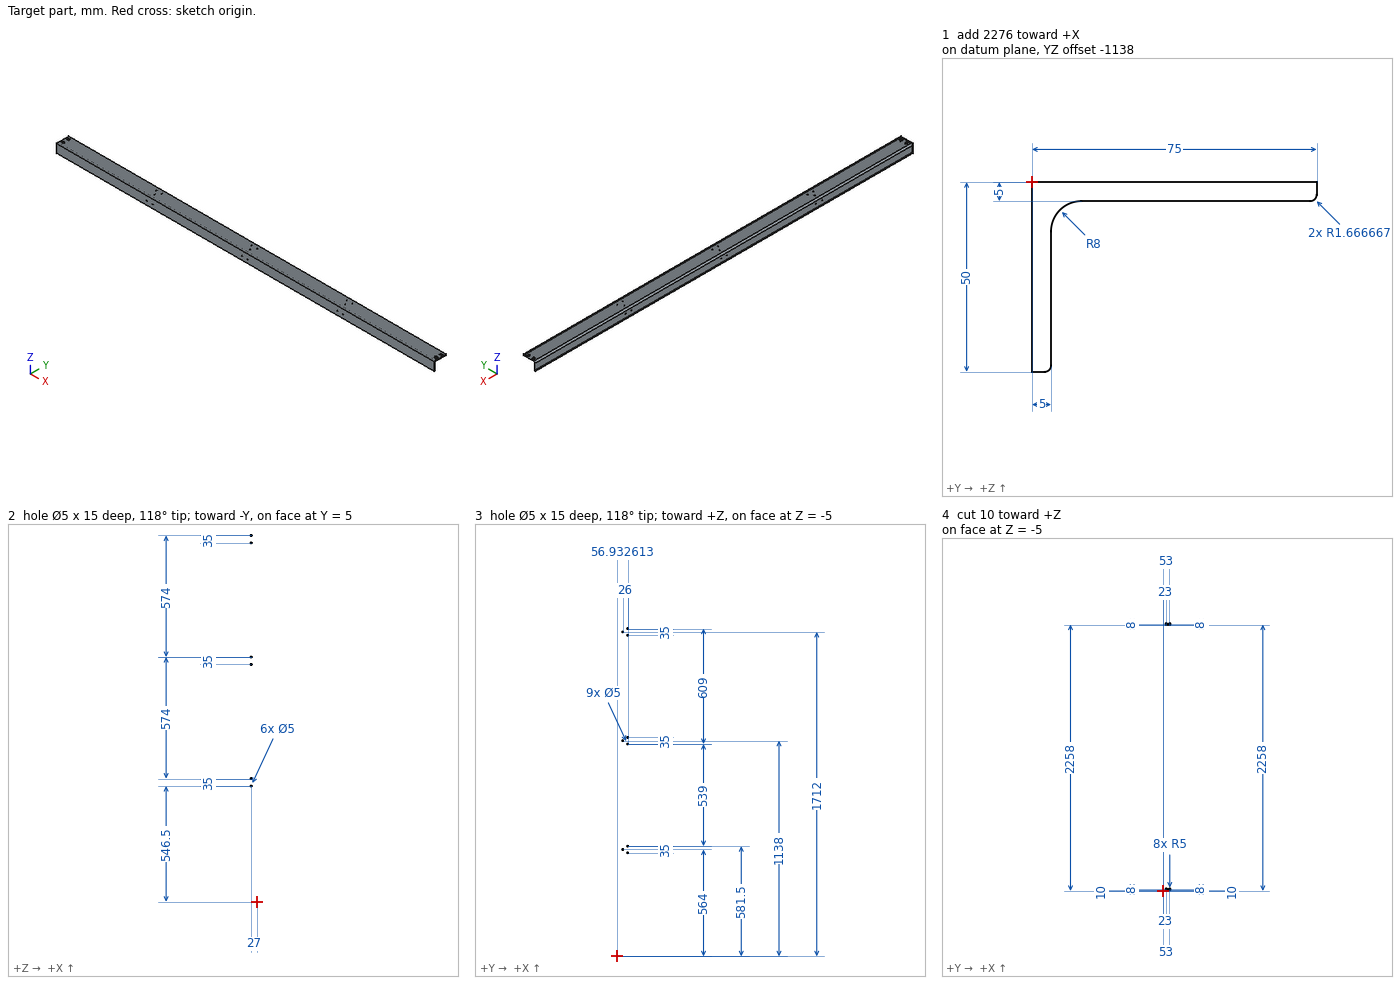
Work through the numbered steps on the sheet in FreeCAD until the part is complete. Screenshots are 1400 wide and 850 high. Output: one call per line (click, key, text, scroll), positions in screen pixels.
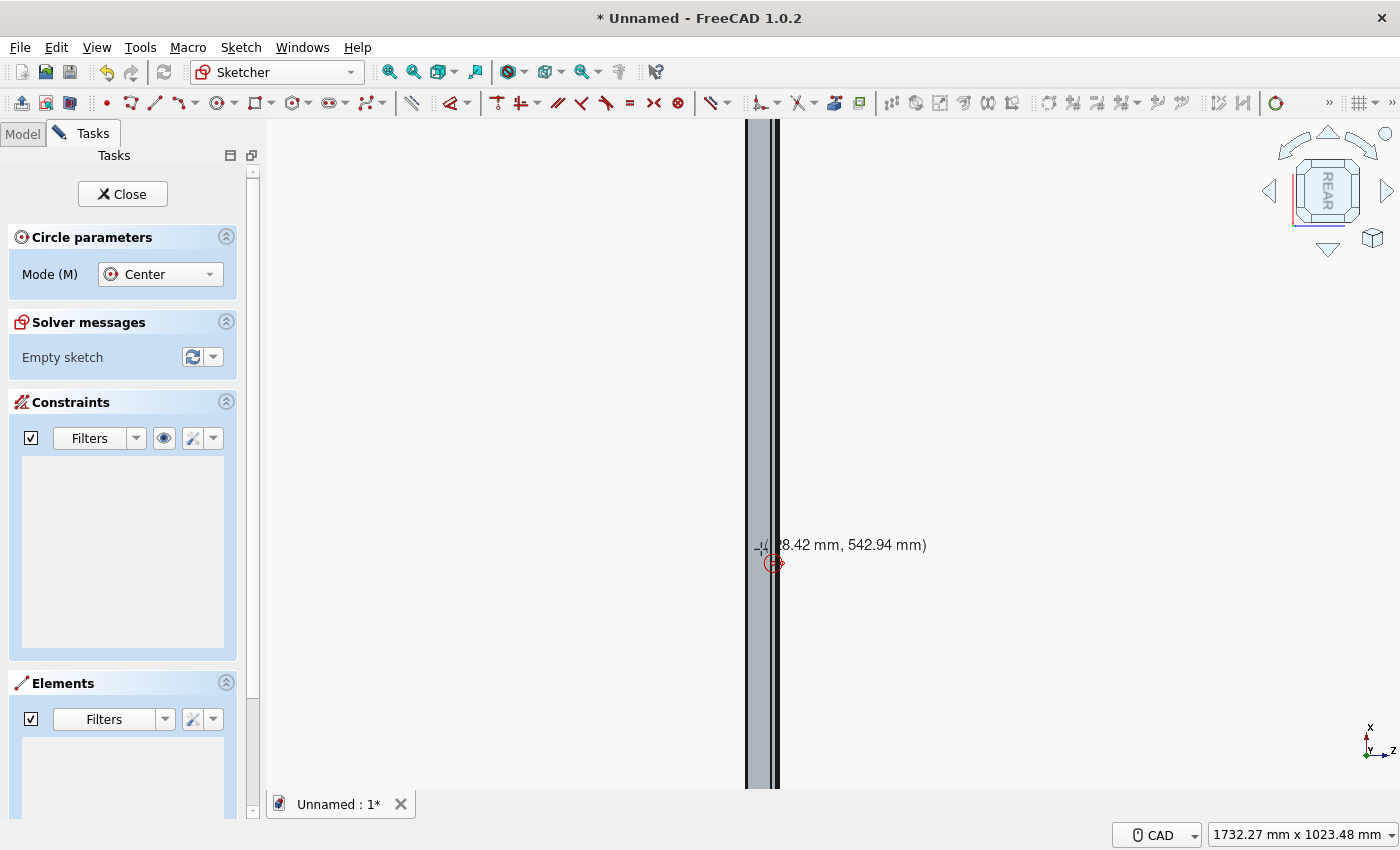
click(761, 548)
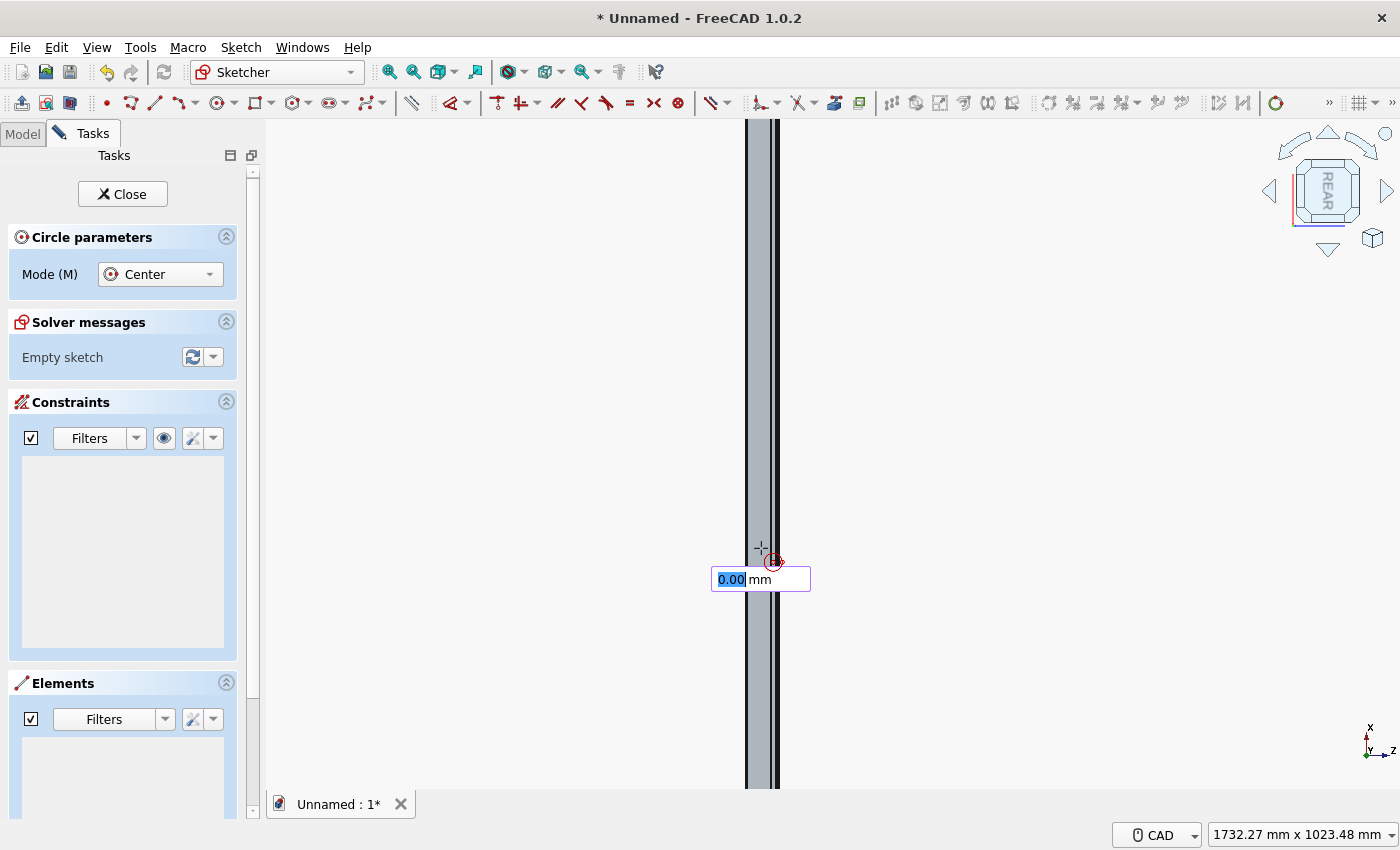
scroll(763, 547, up, 12)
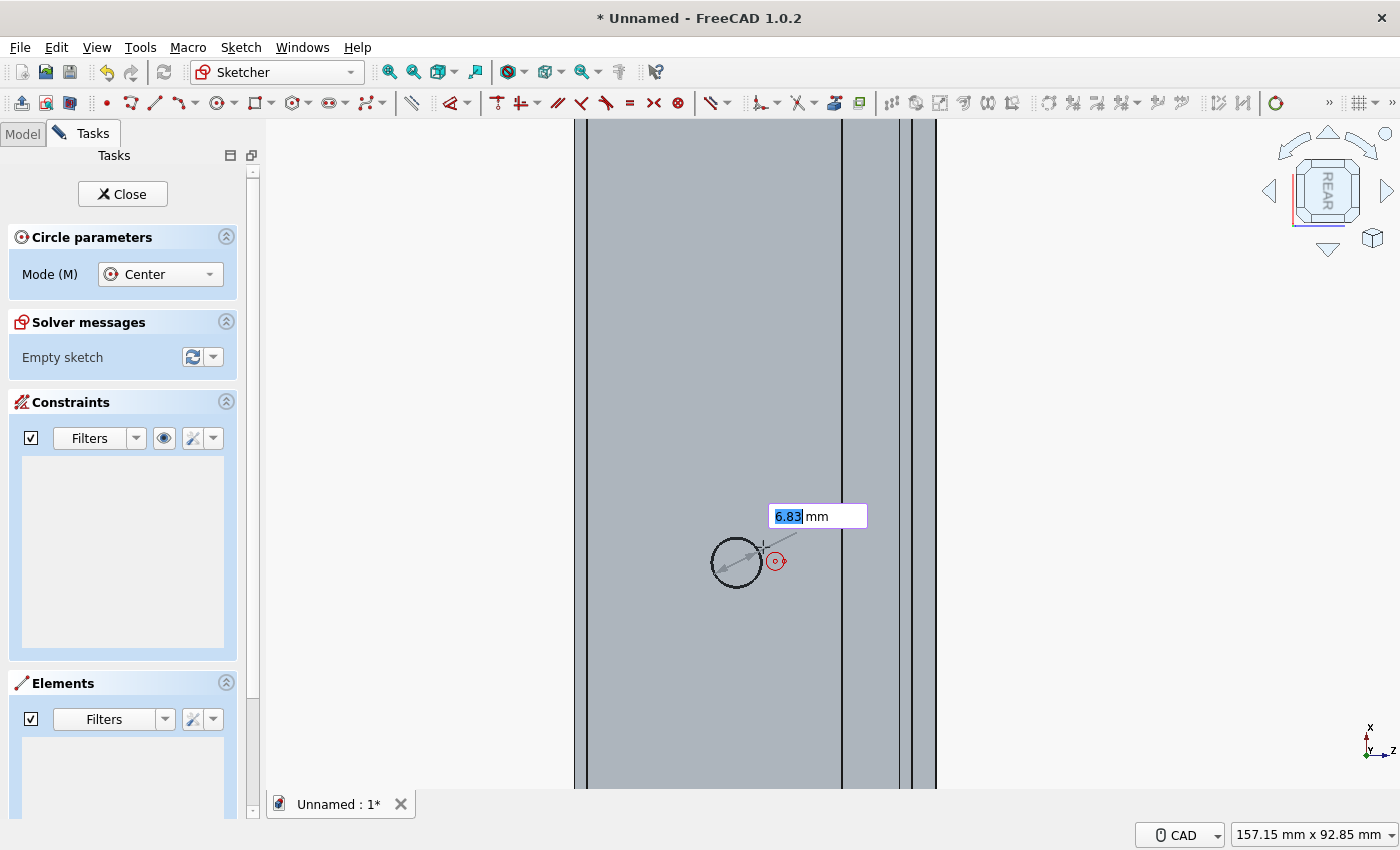
click(754, 540)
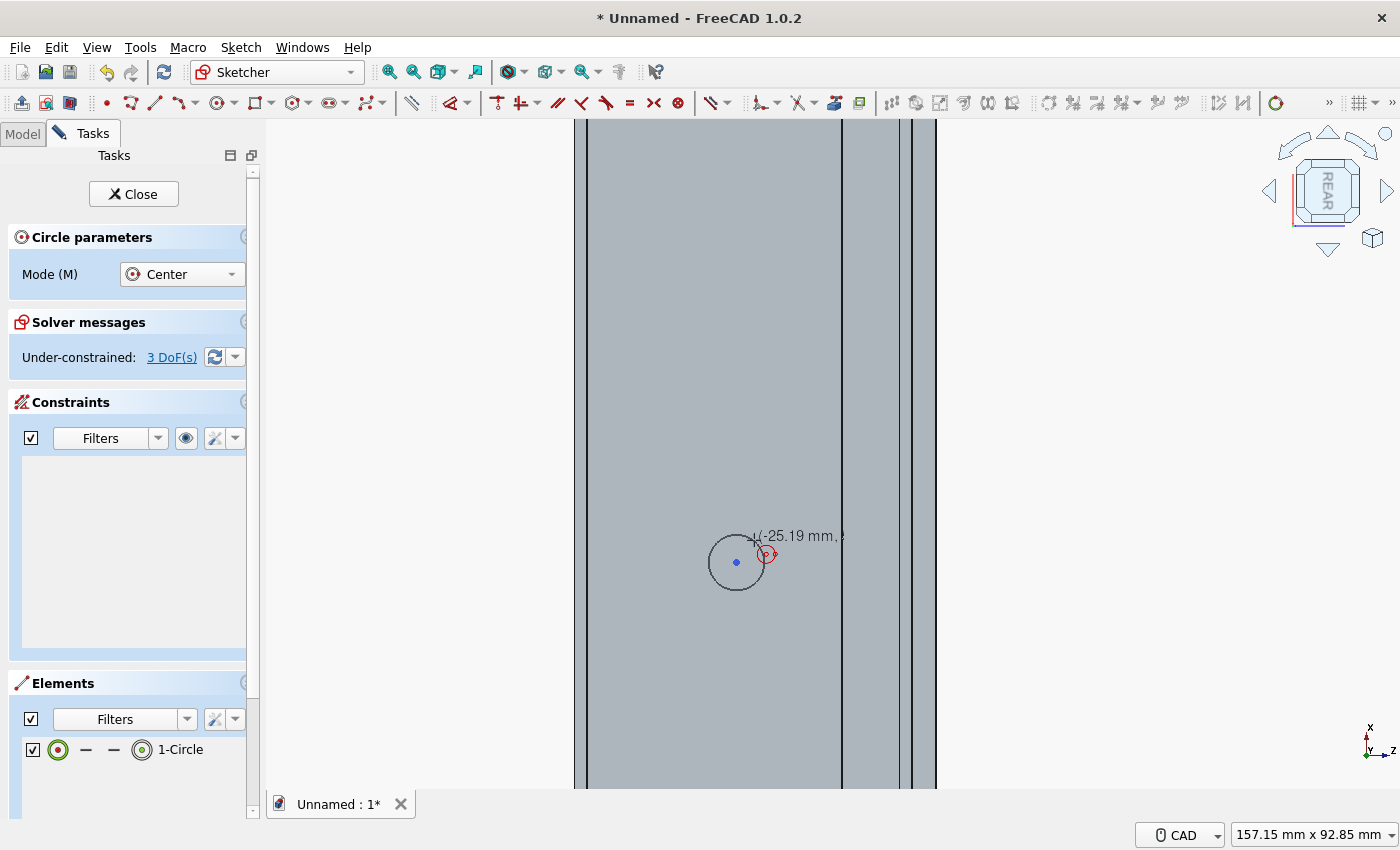
scroll(741, 300, up, 2)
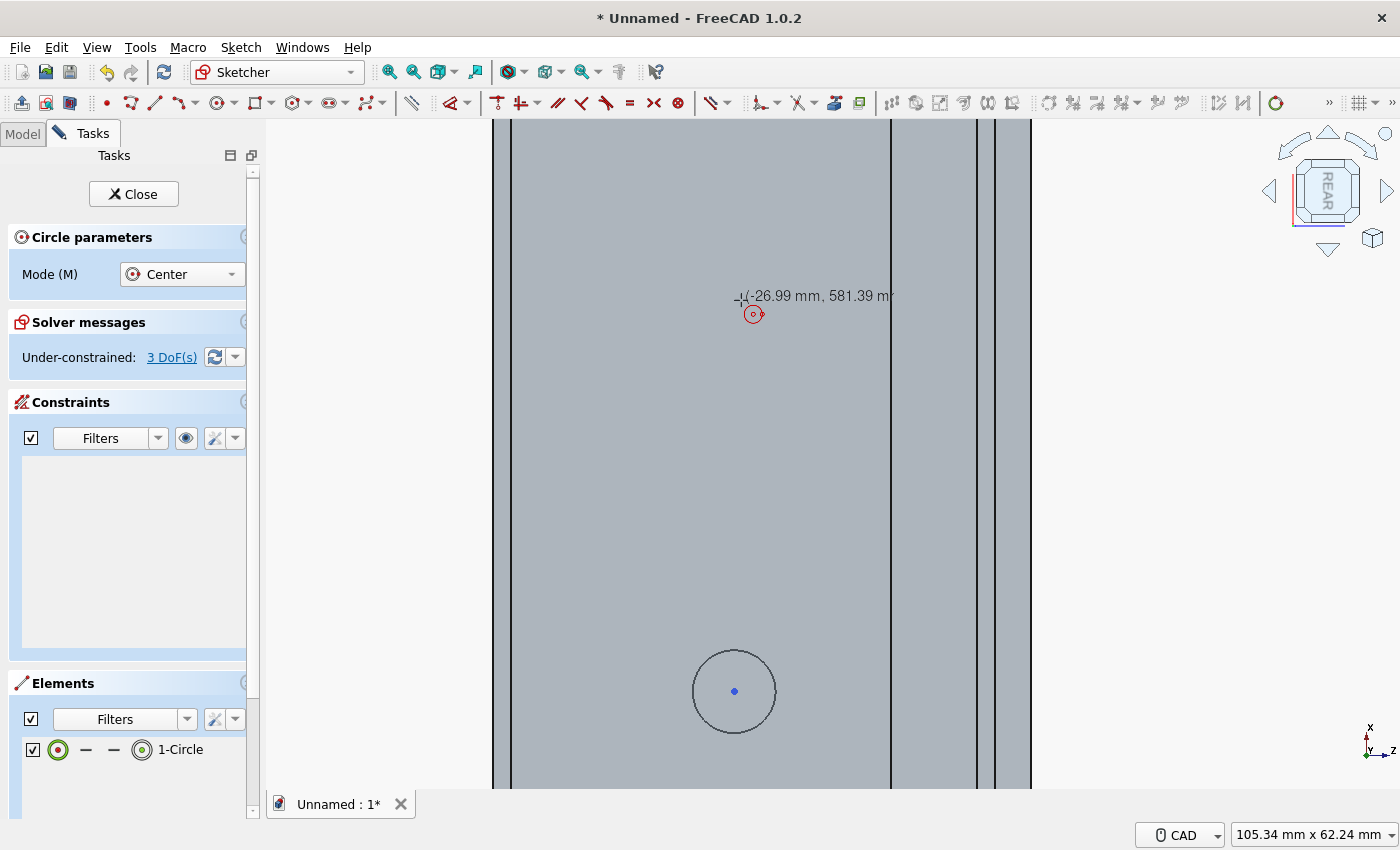
scroll(761, 544, down, 18)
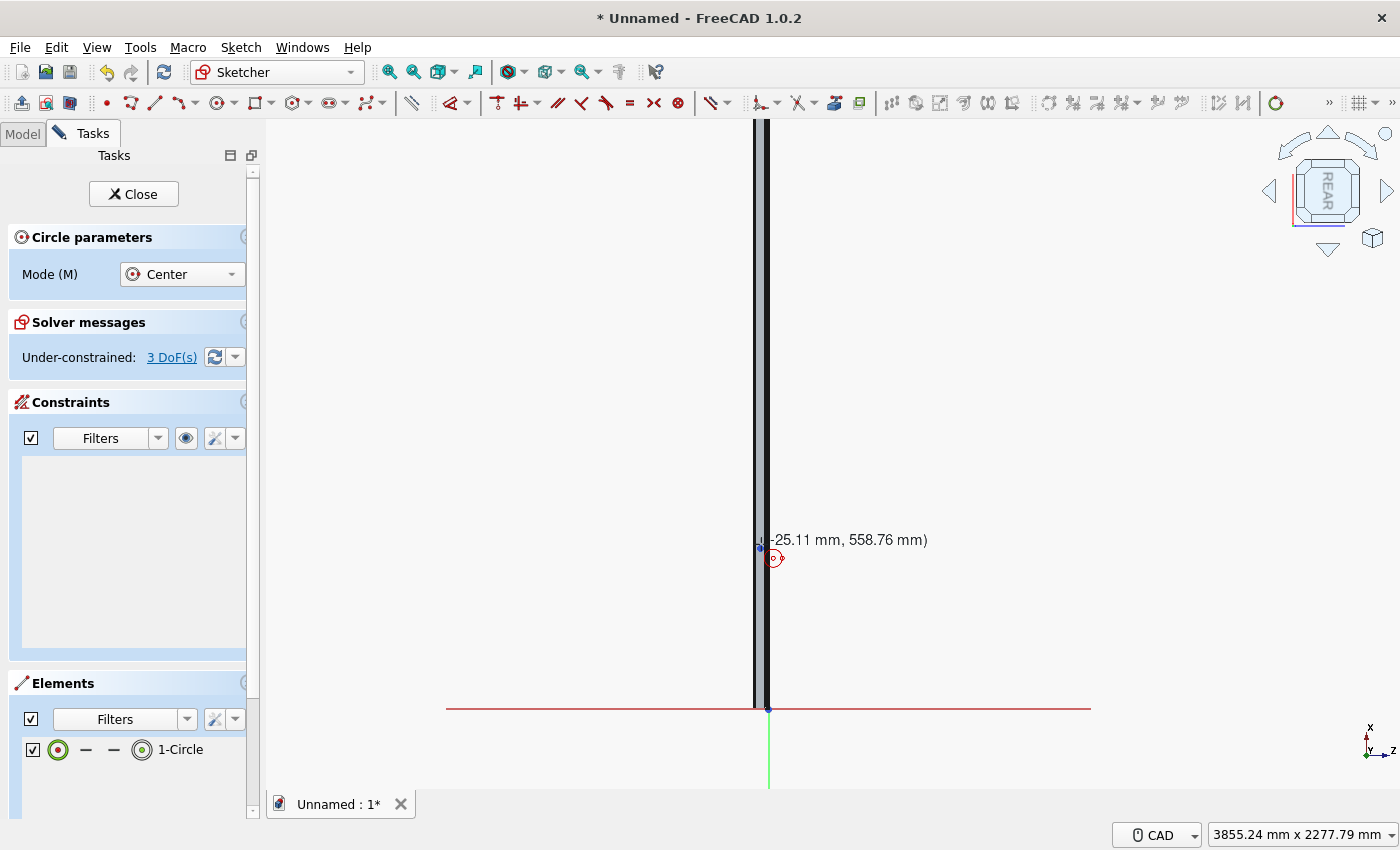
scroll(761, 538, up, 4)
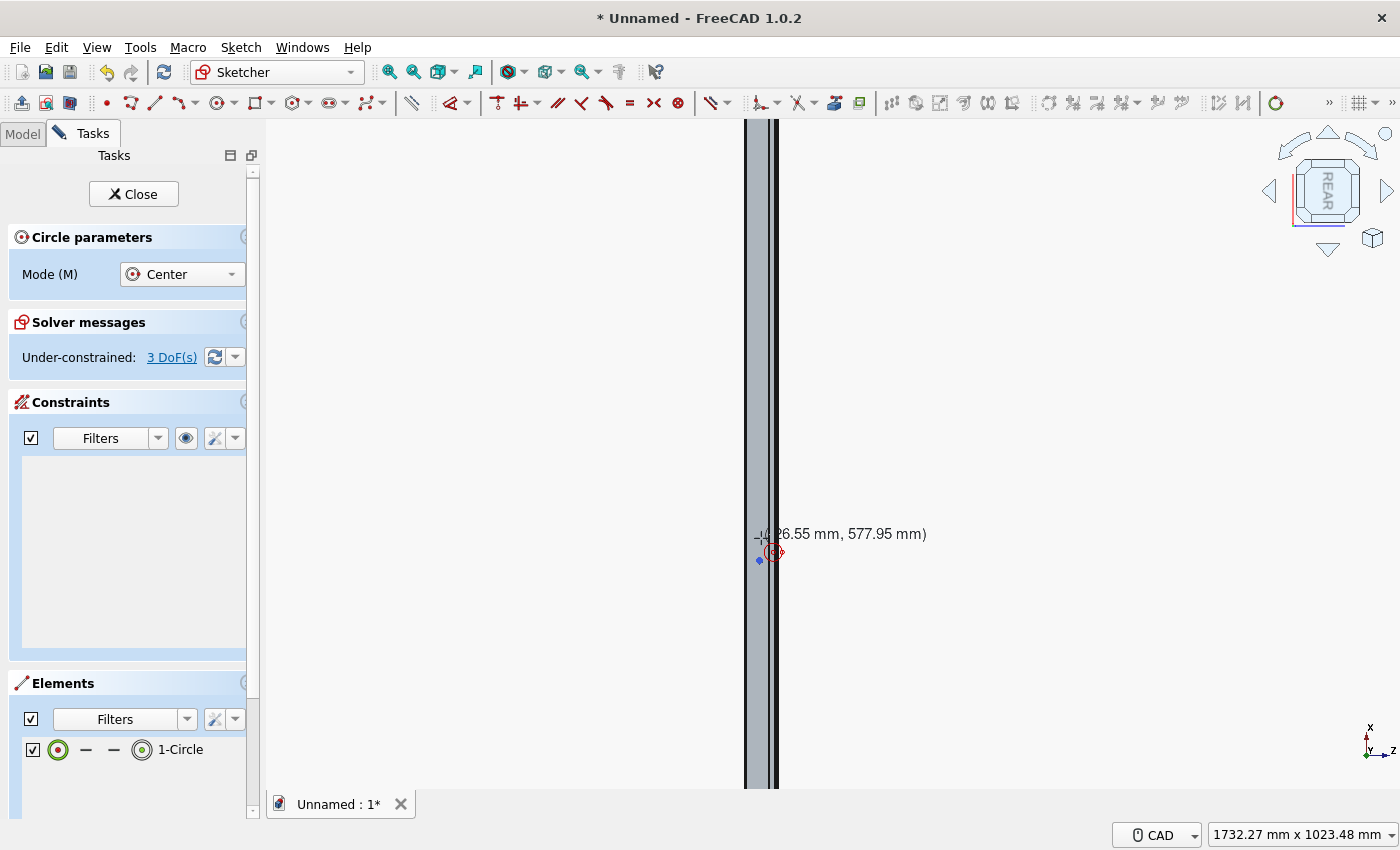
click(760, 537)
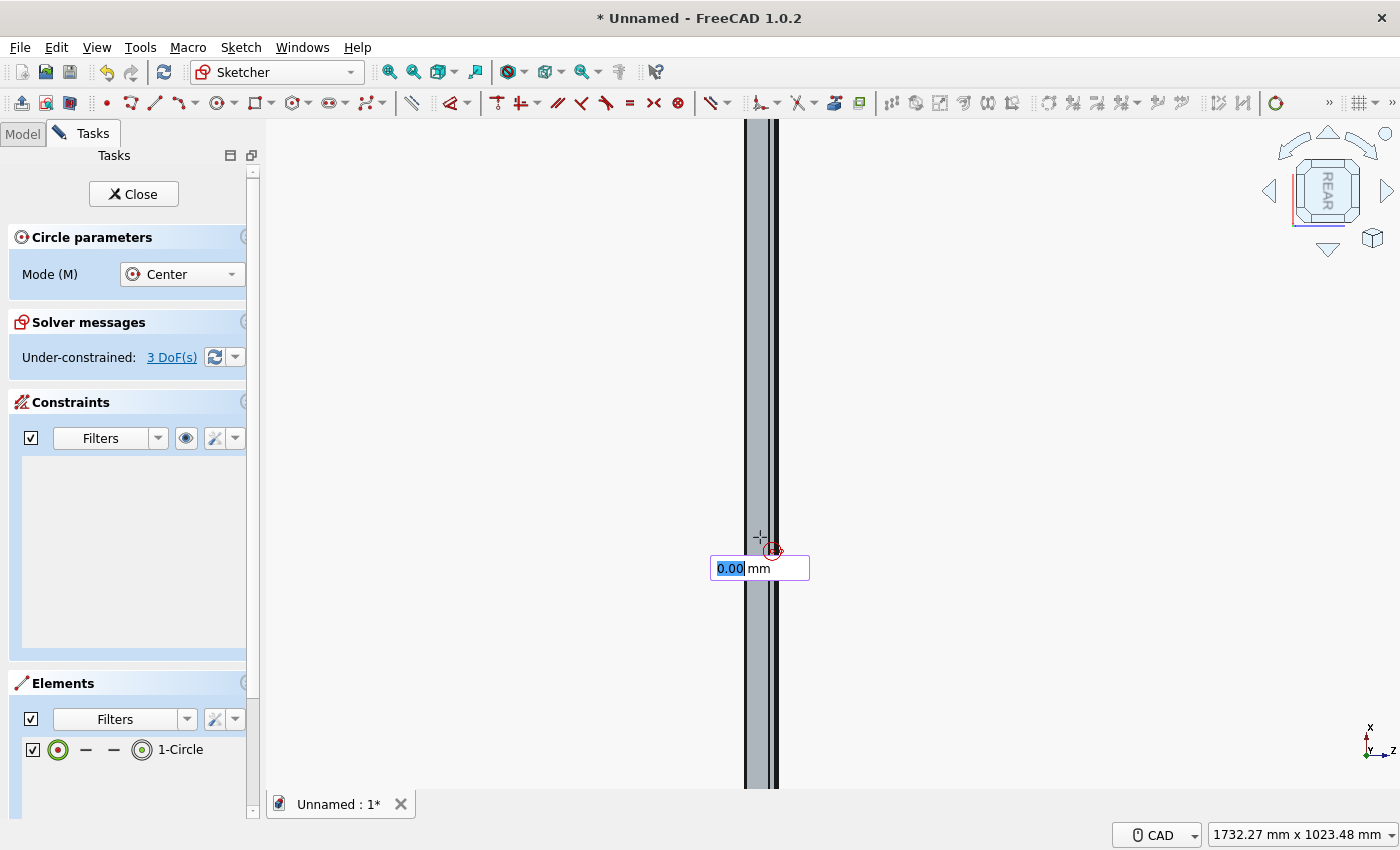
scroll(761, 536, up, 12)